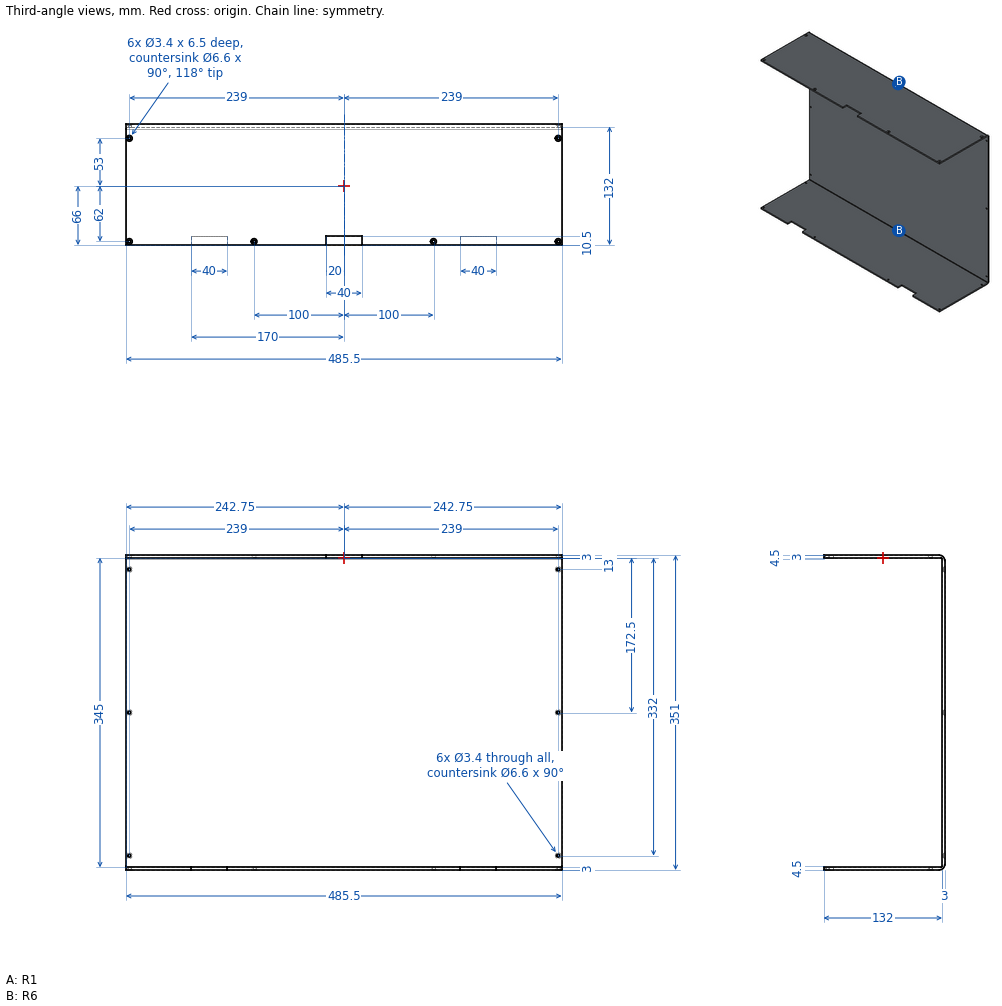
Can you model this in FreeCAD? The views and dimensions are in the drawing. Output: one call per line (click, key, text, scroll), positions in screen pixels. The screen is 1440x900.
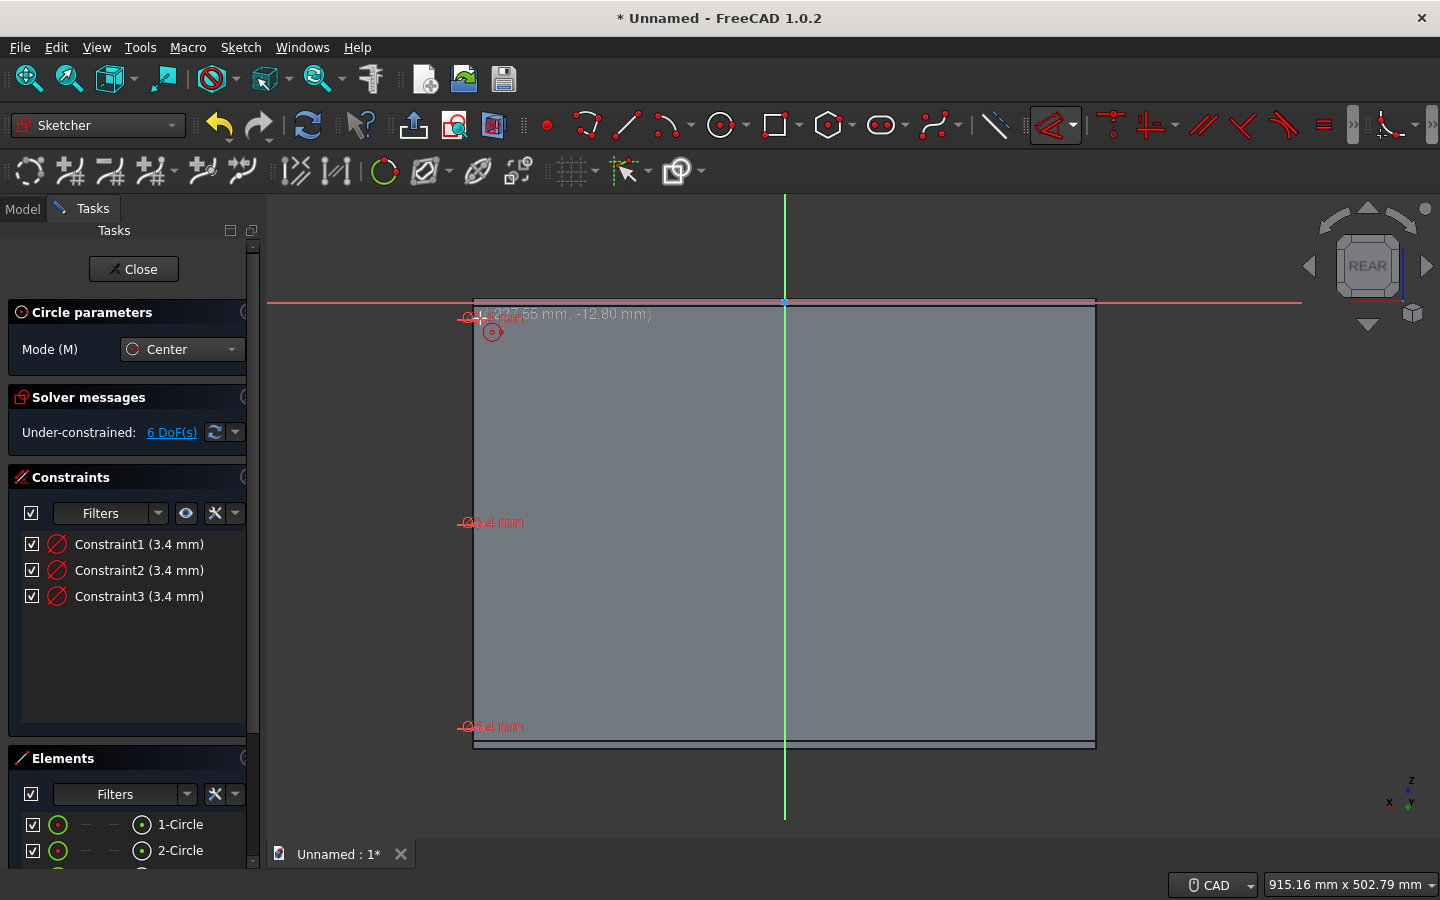
scroll(1091, 728, up, 12)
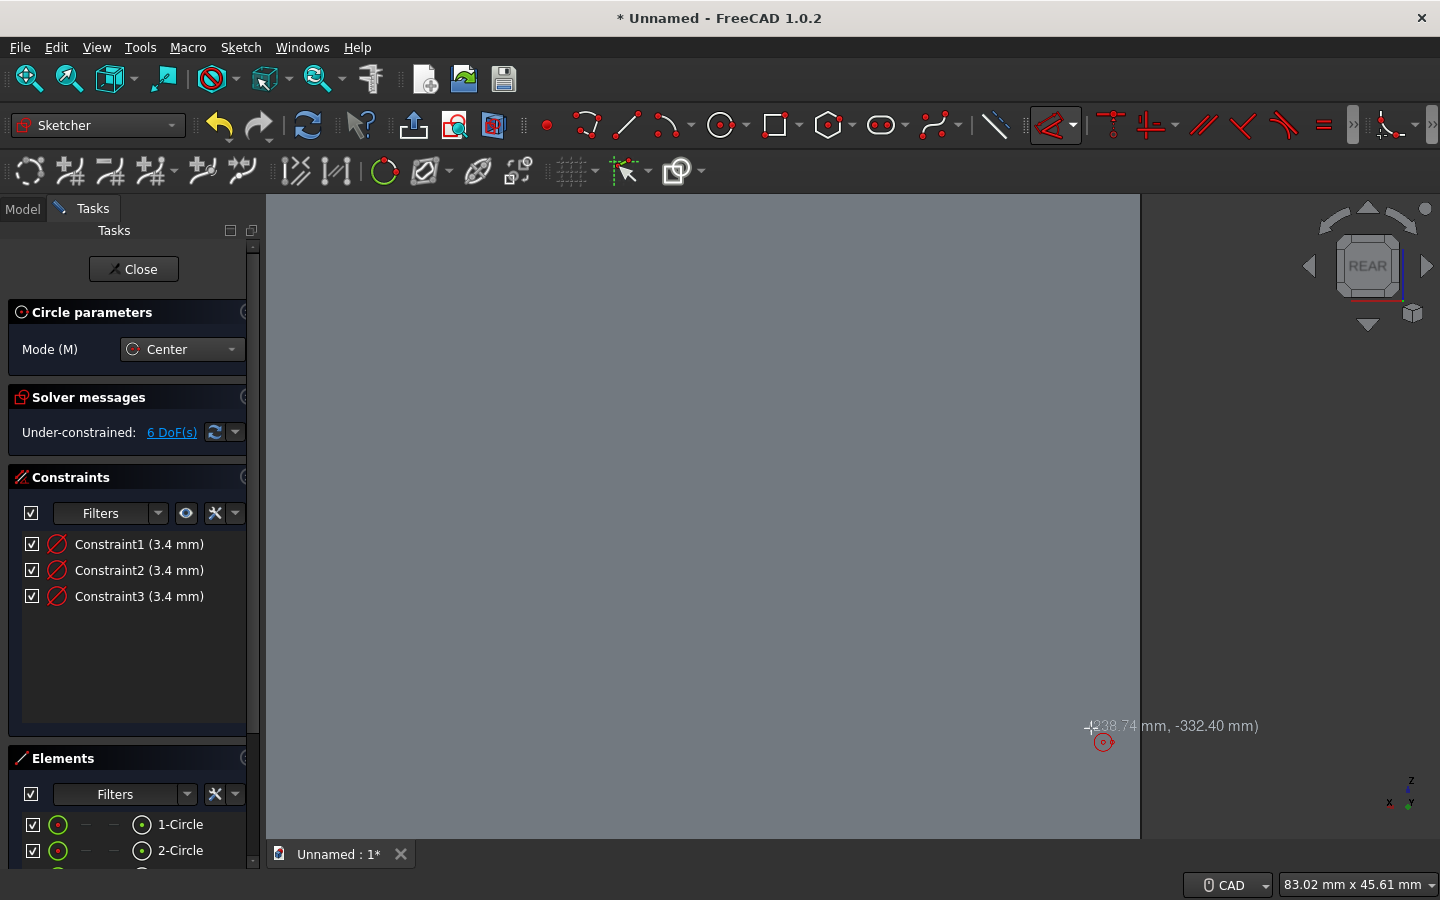
scroll(1091, 729, down, 12)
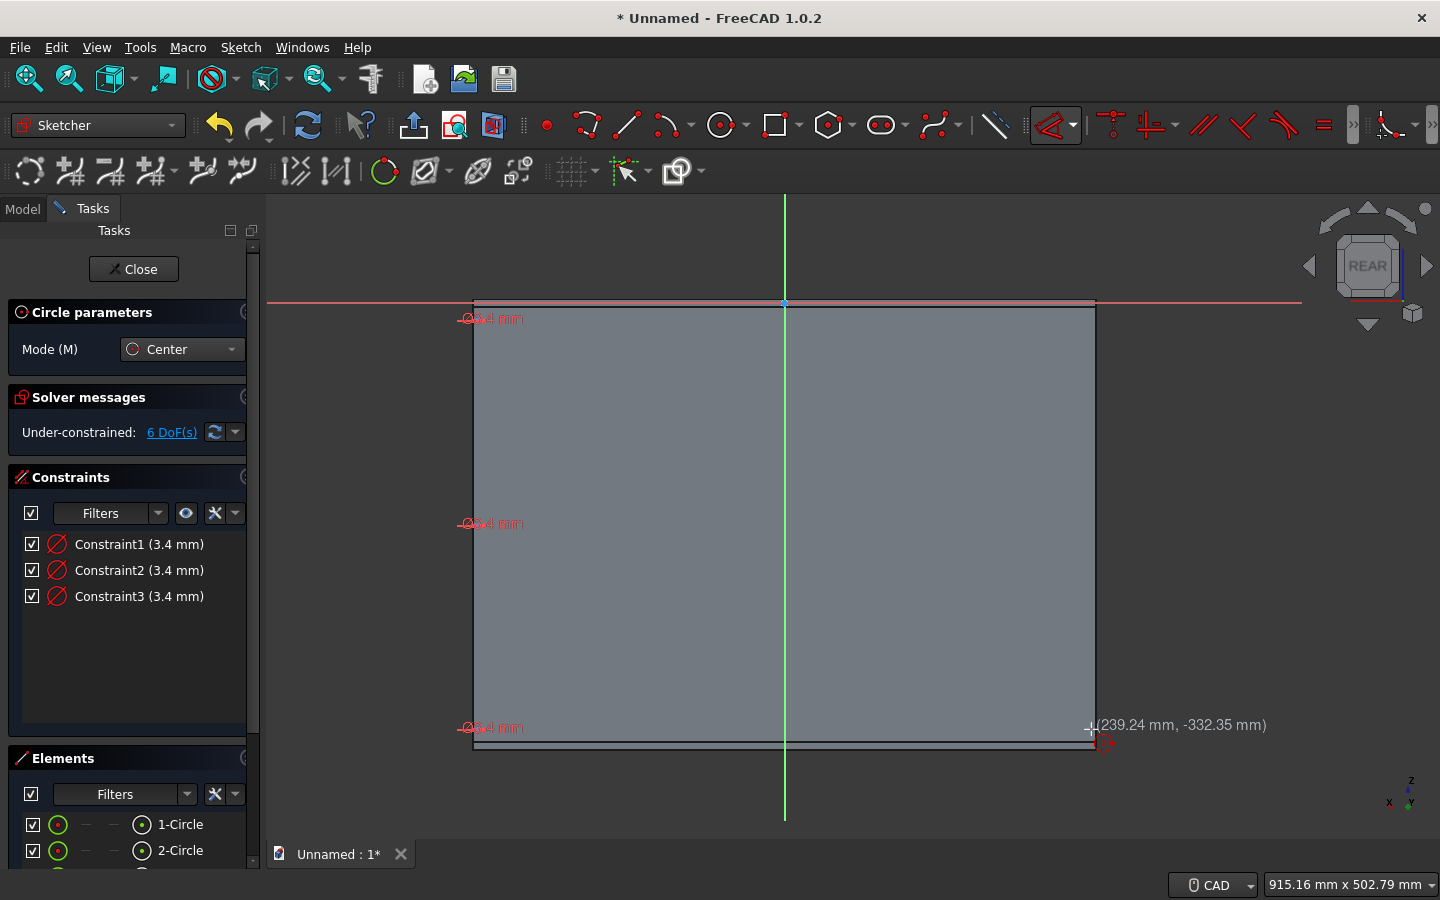
click(1091, 729)
move(1093, 728)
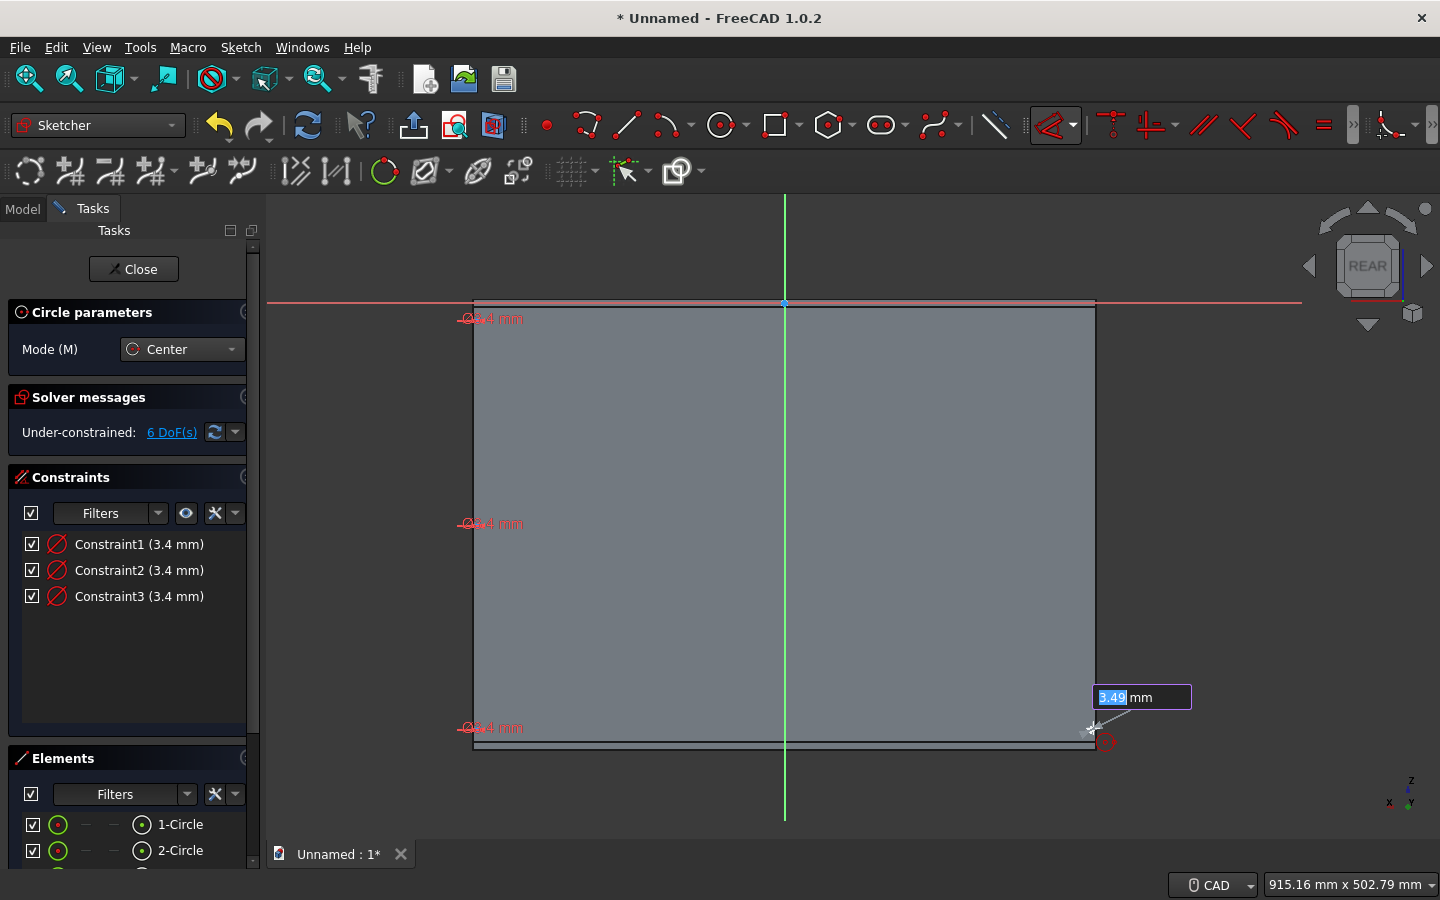
text(3.4)
key(Return)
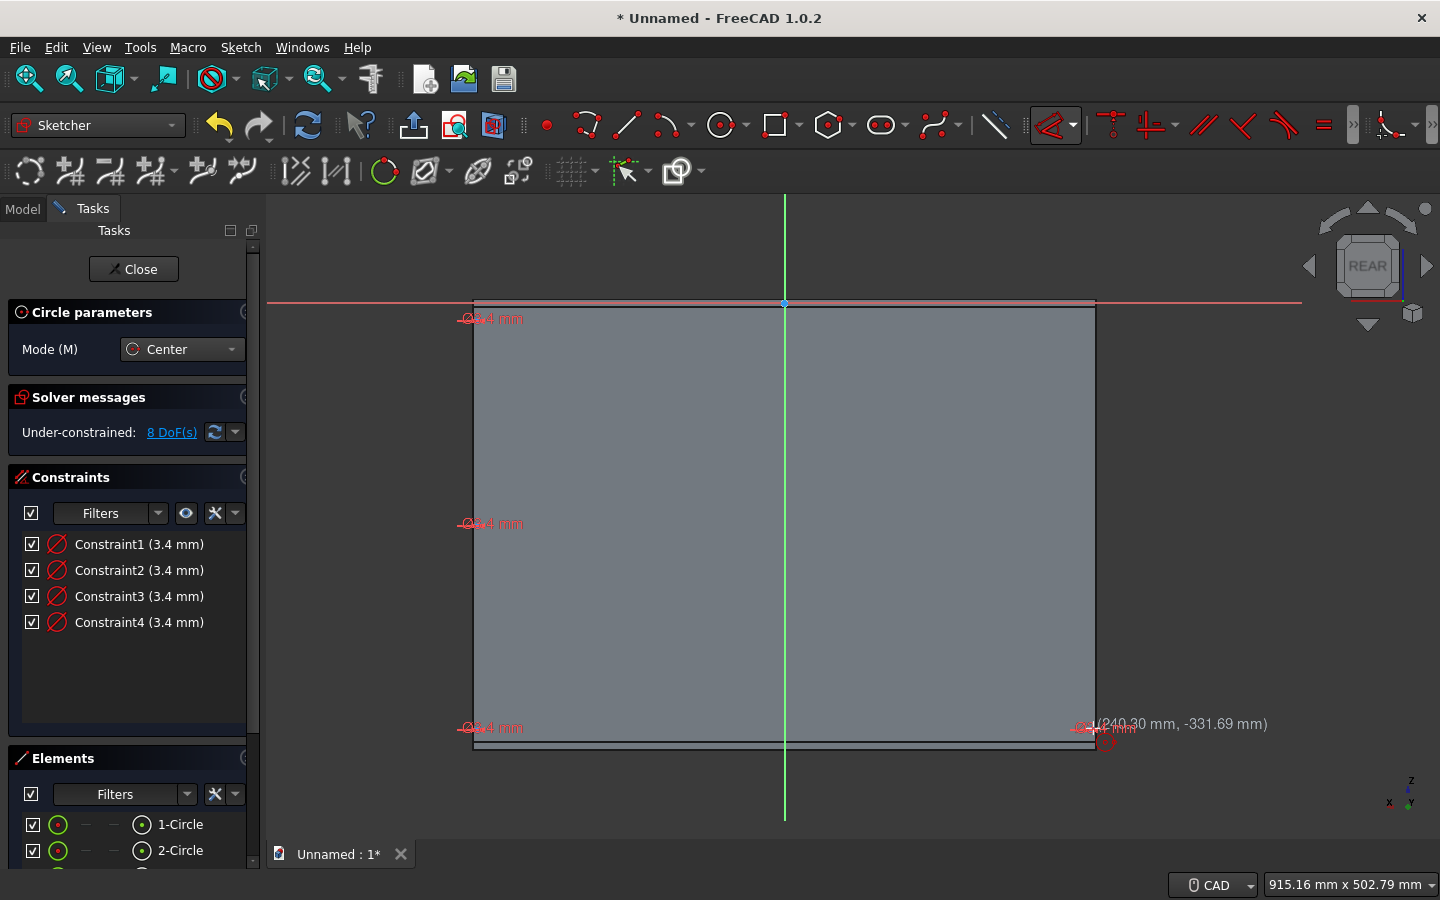
scroll(1091, 525, up, 12)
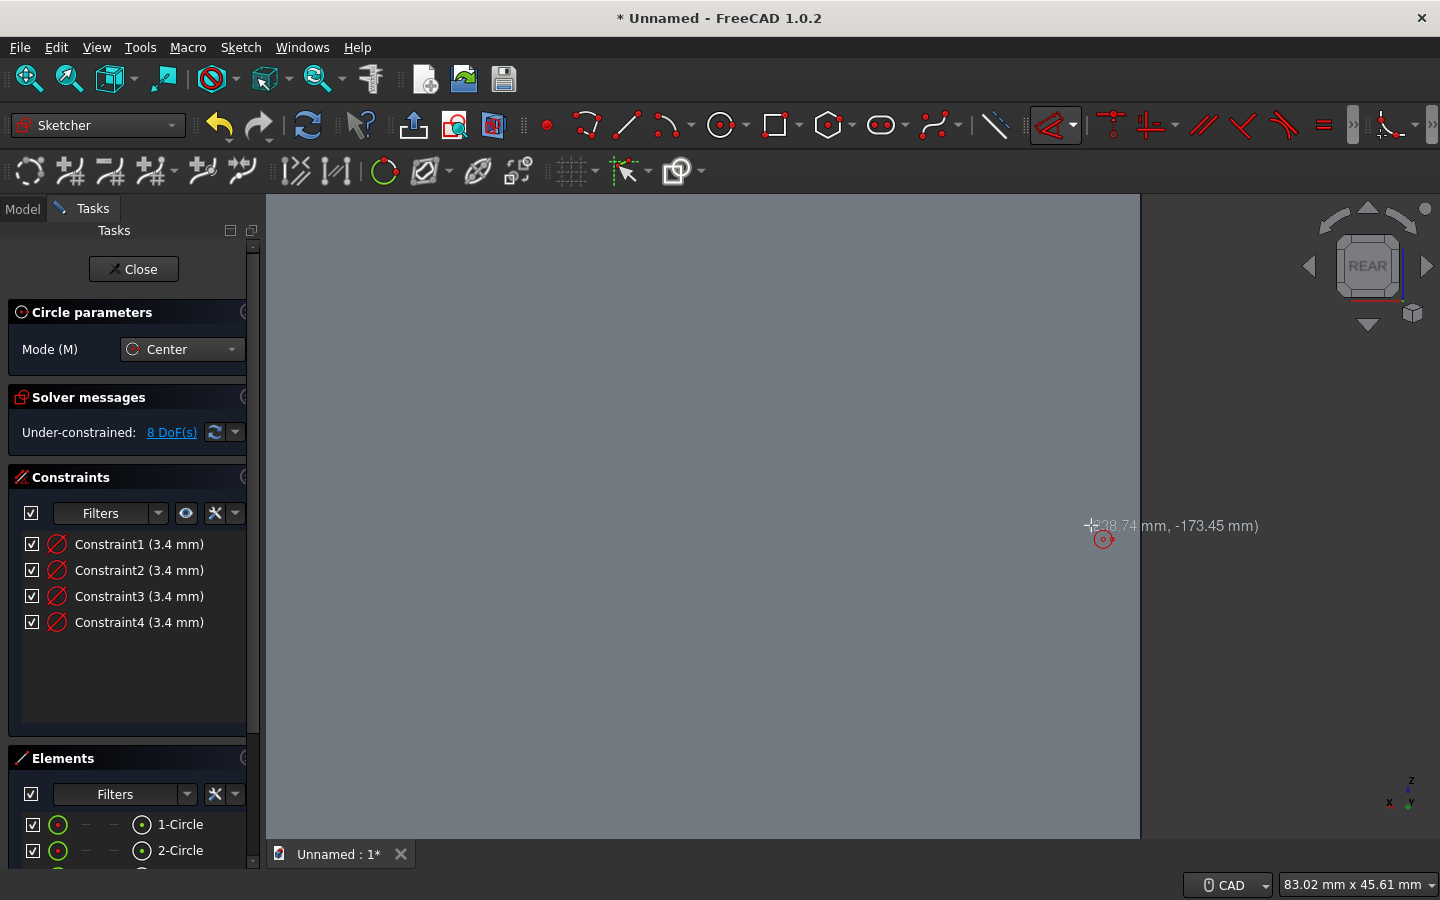
scroll(1091, 524, down, 12)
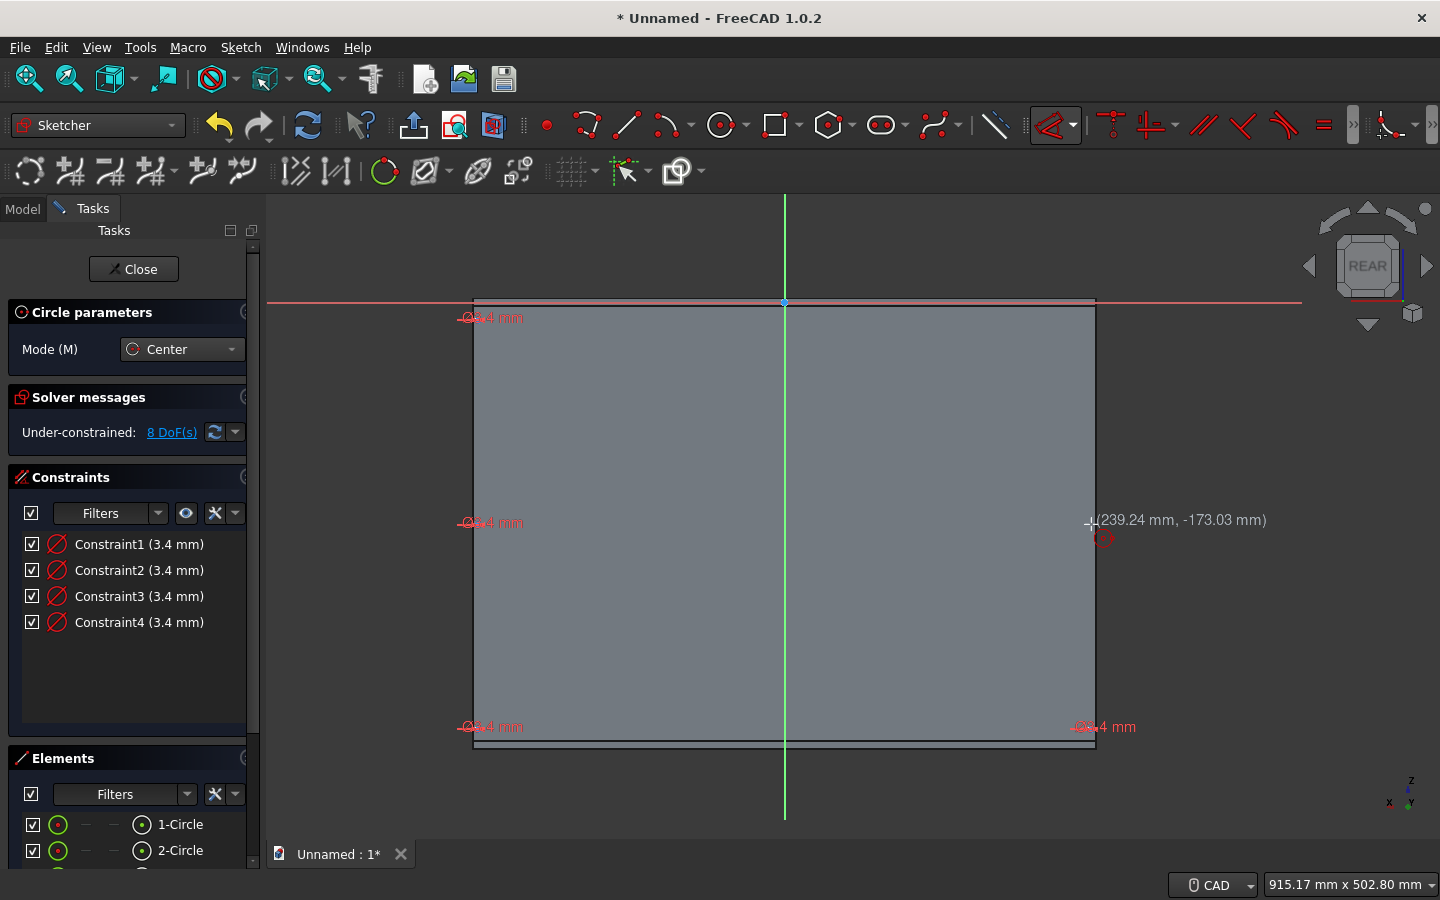
click(1091, 524)
move(1093, 522)